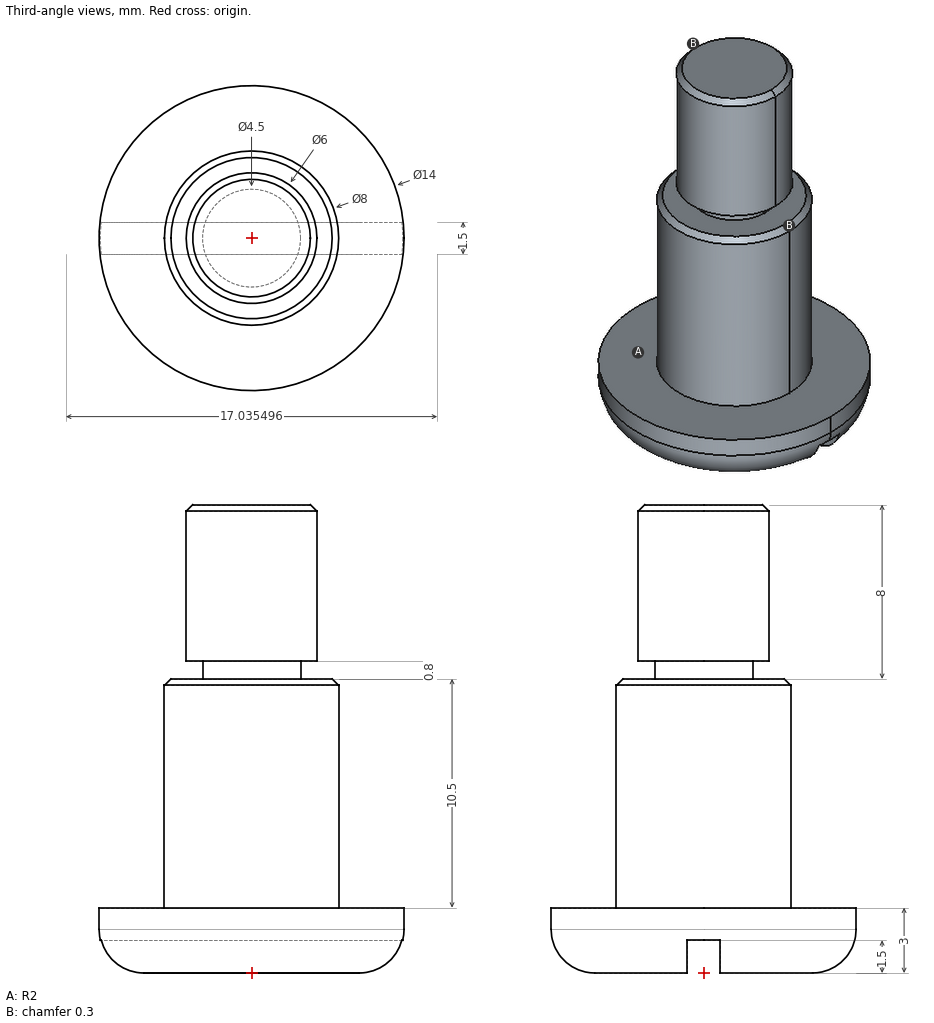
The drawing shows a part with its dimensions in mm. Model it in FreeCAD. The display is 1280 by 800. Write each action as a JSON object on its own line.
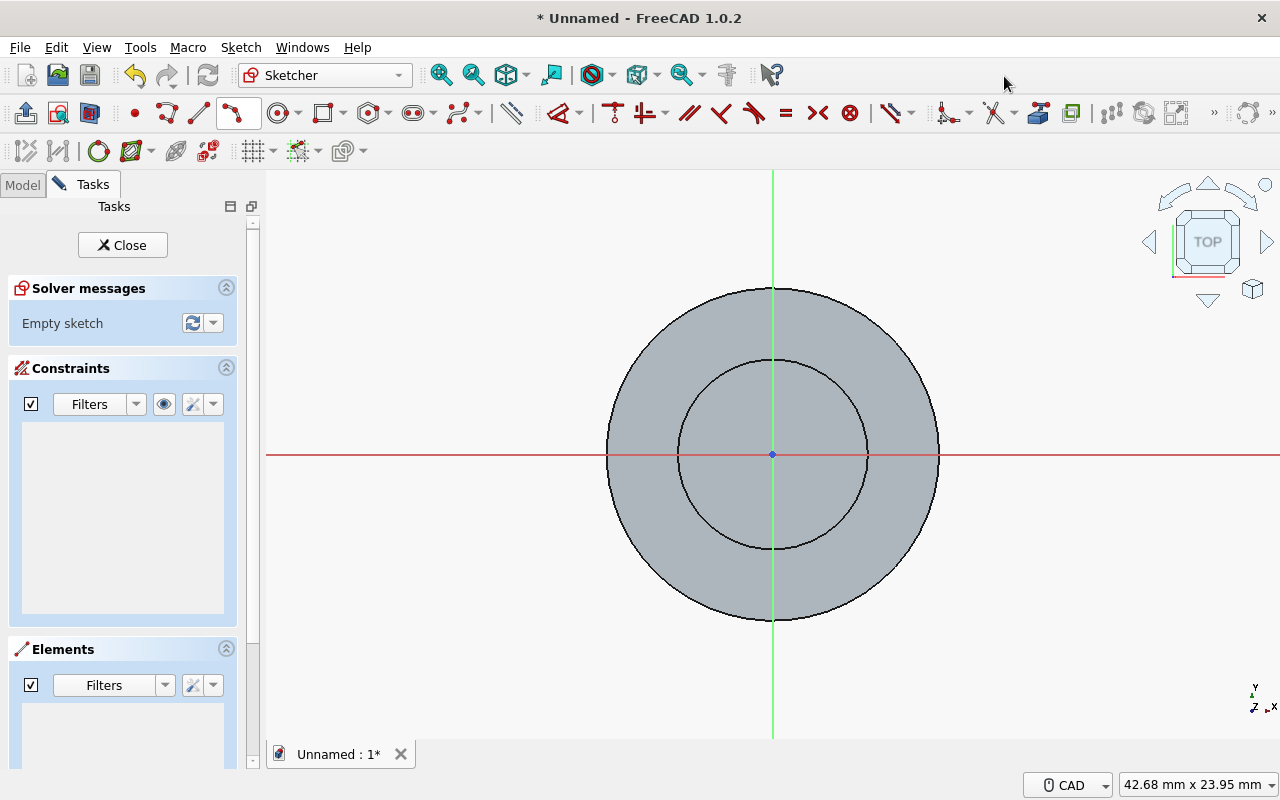
{"action": "scroll", "coordinate": [813, 454], "scroll_direction": "up", "scroll_amount": 5}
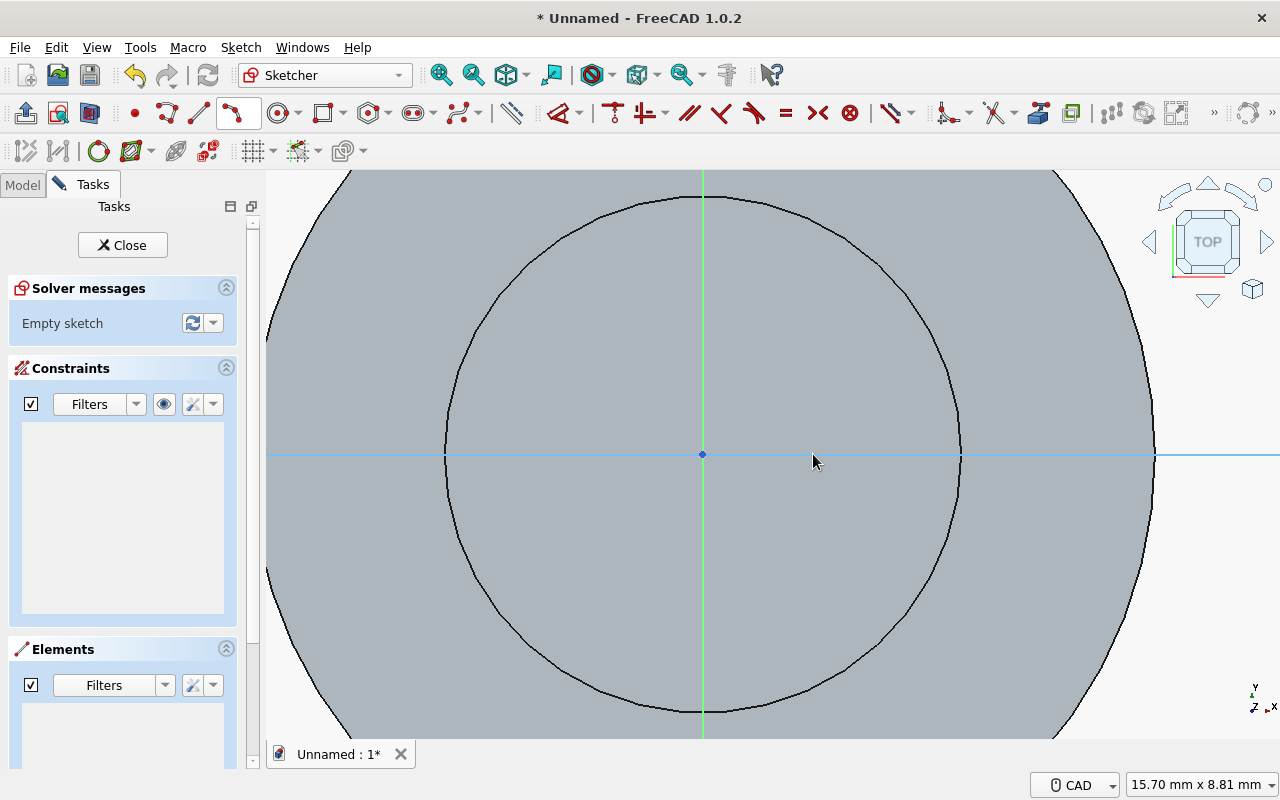
{"action": "left_click", "coordinate": [278, 114]}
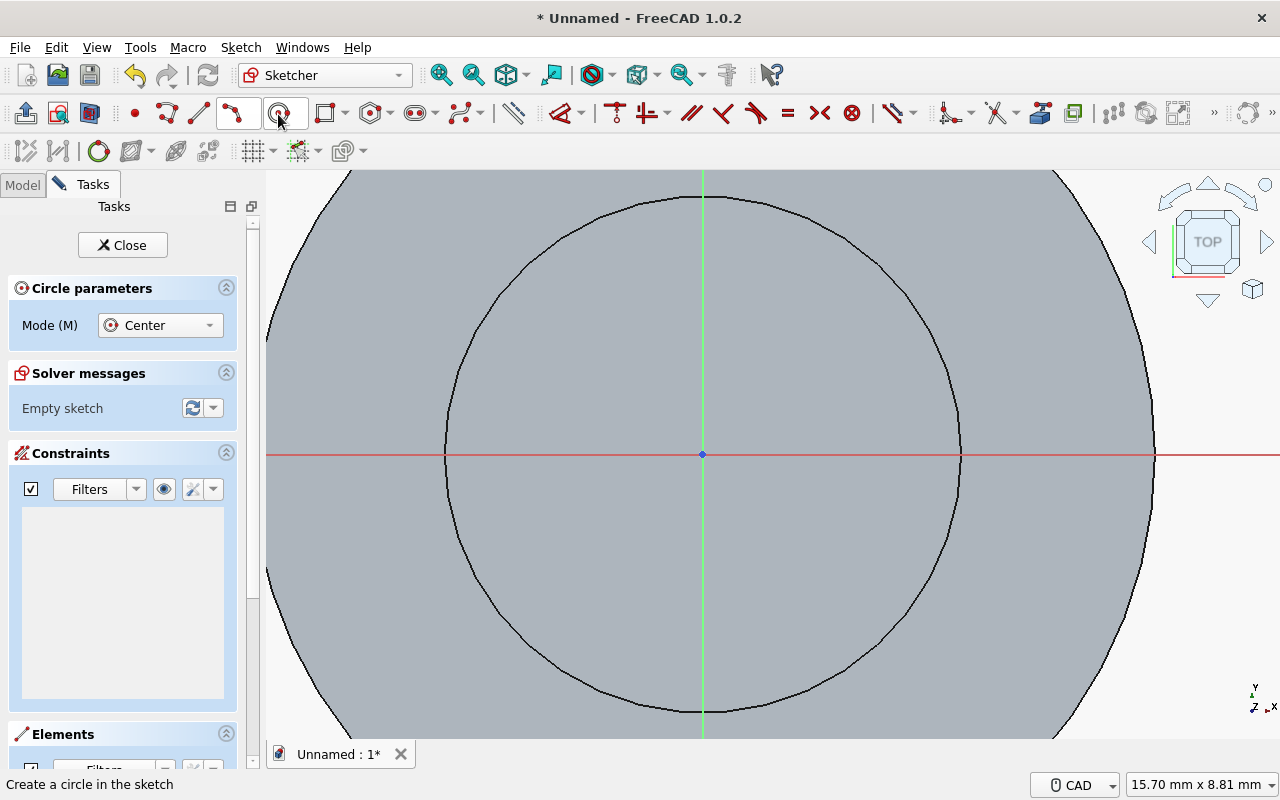
{"action": "left_click", "coordinate": [703, 454]}
{"action": "left_click", "coordinate": [840, 318]}
{"action": "key", "text": "Escape"}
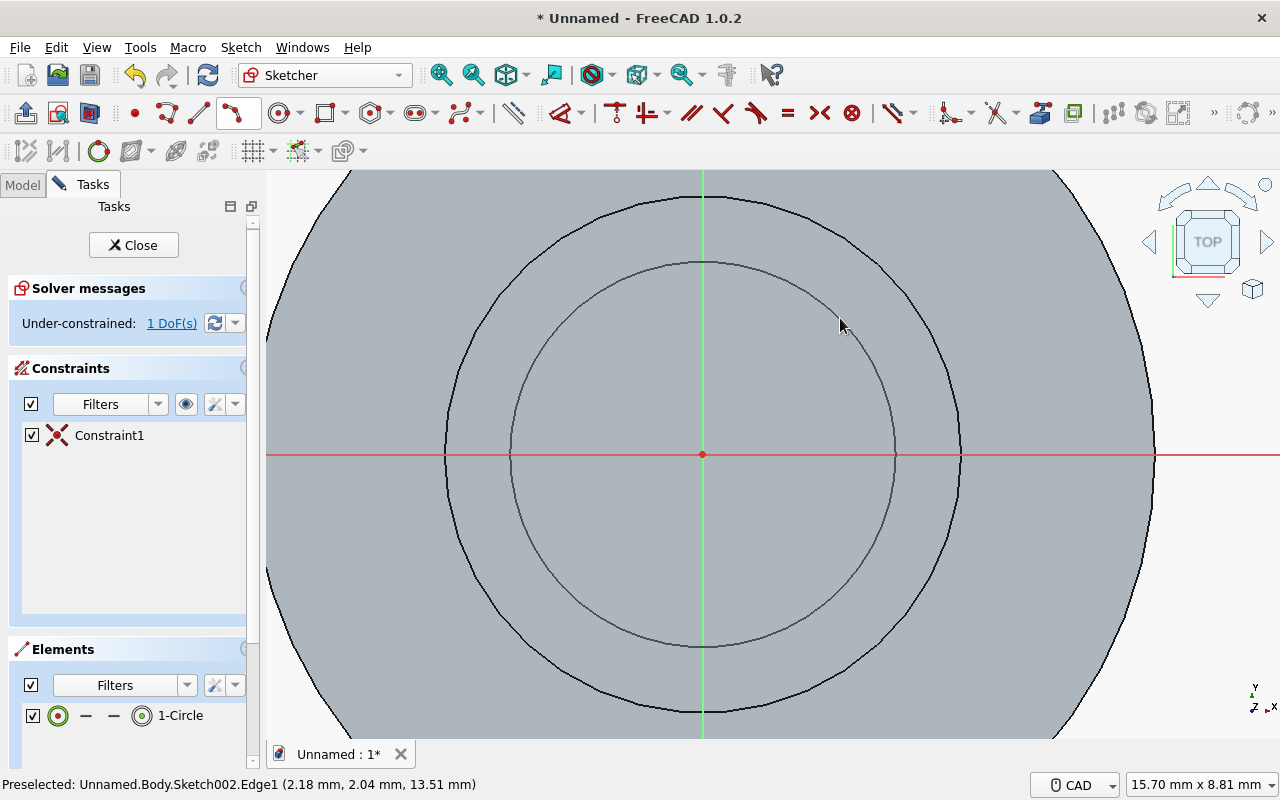
{"action": "key", "text": "d"}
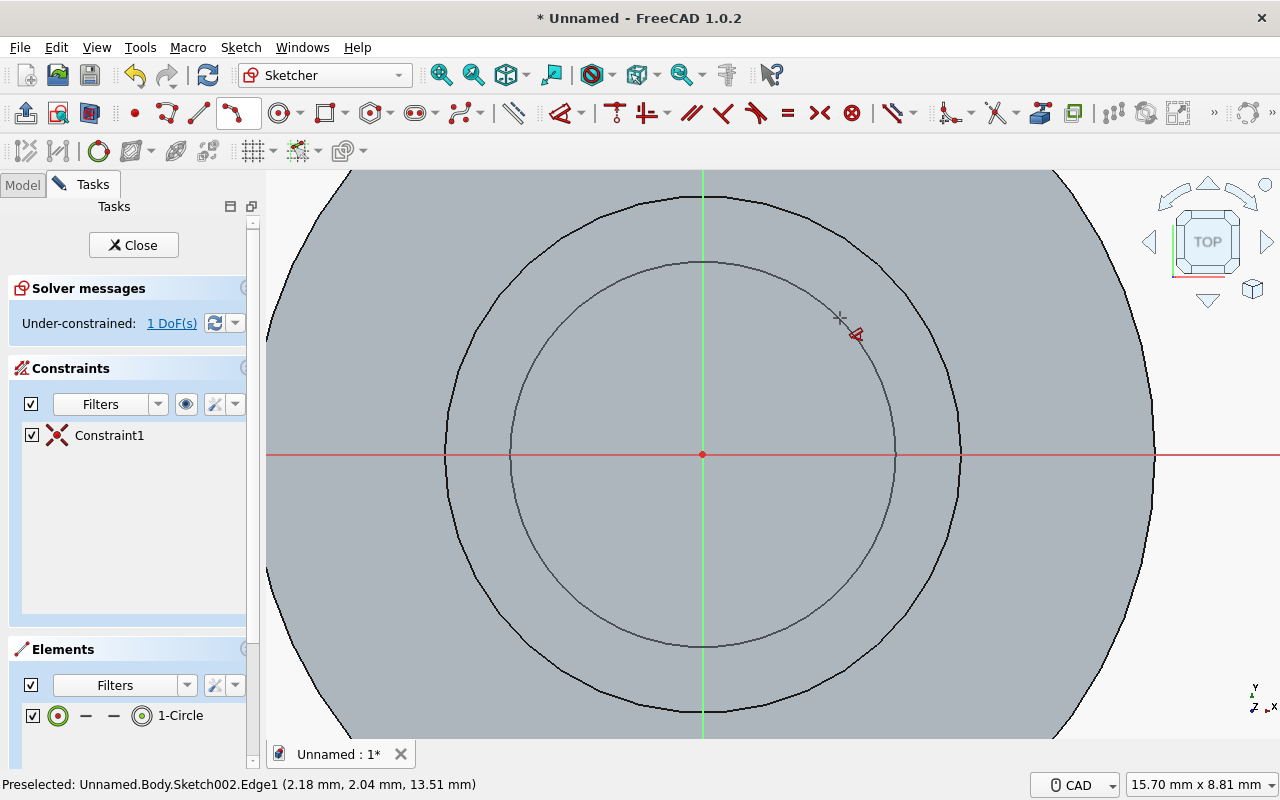
{"action": "left_click", "coordinate": [839, 318]}
{"action": "left_click", "coordinate": [862, 295]}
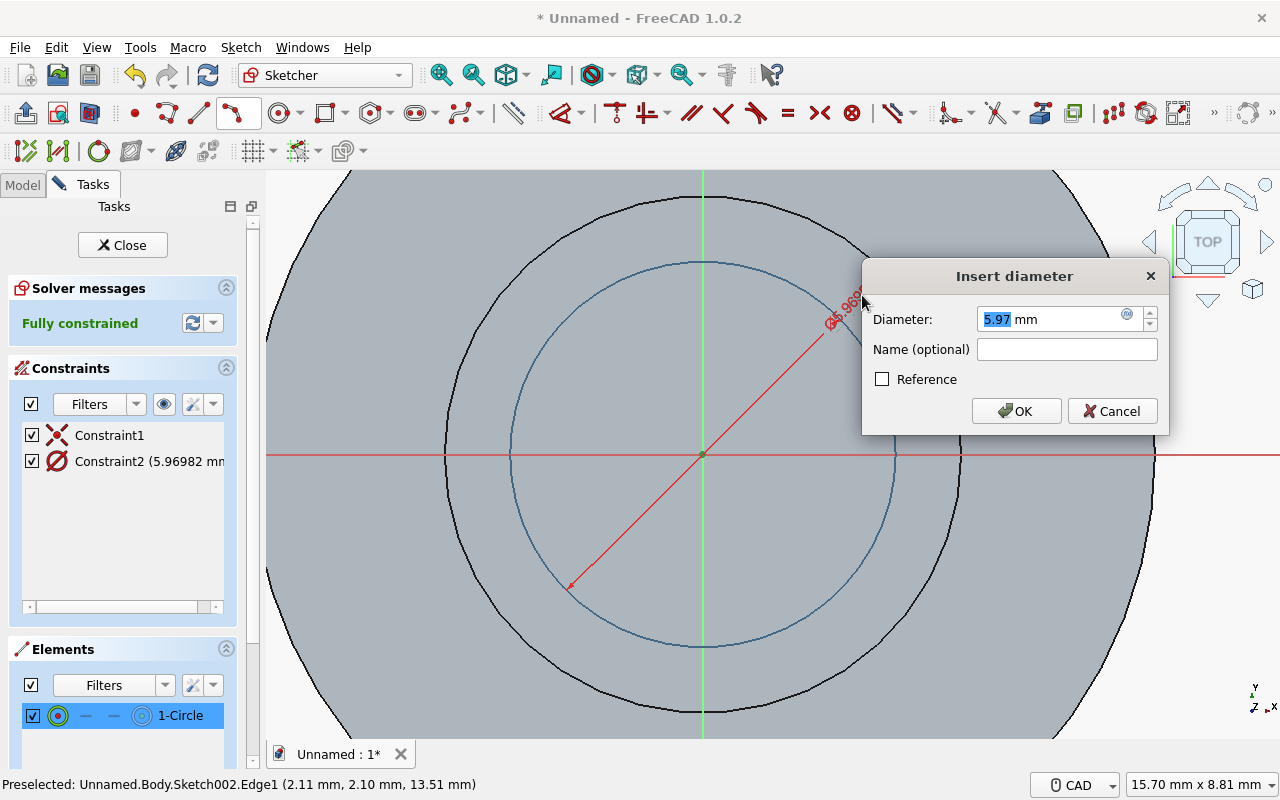
{"action": "type", "text": "6"}
{"action": "key", "text": "Return"}
{"action": "key", "text": "Escape"}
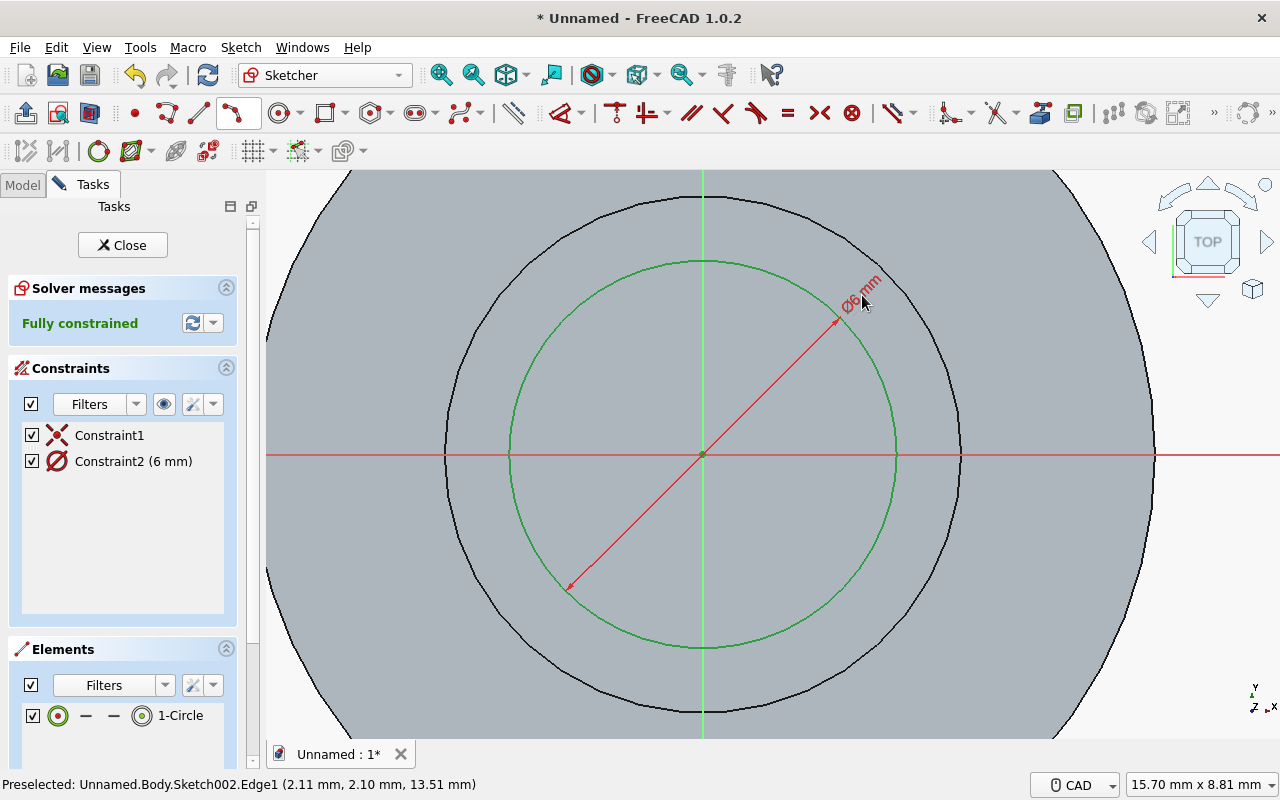
{"action": "left_click", "coordinate": [123, 245]}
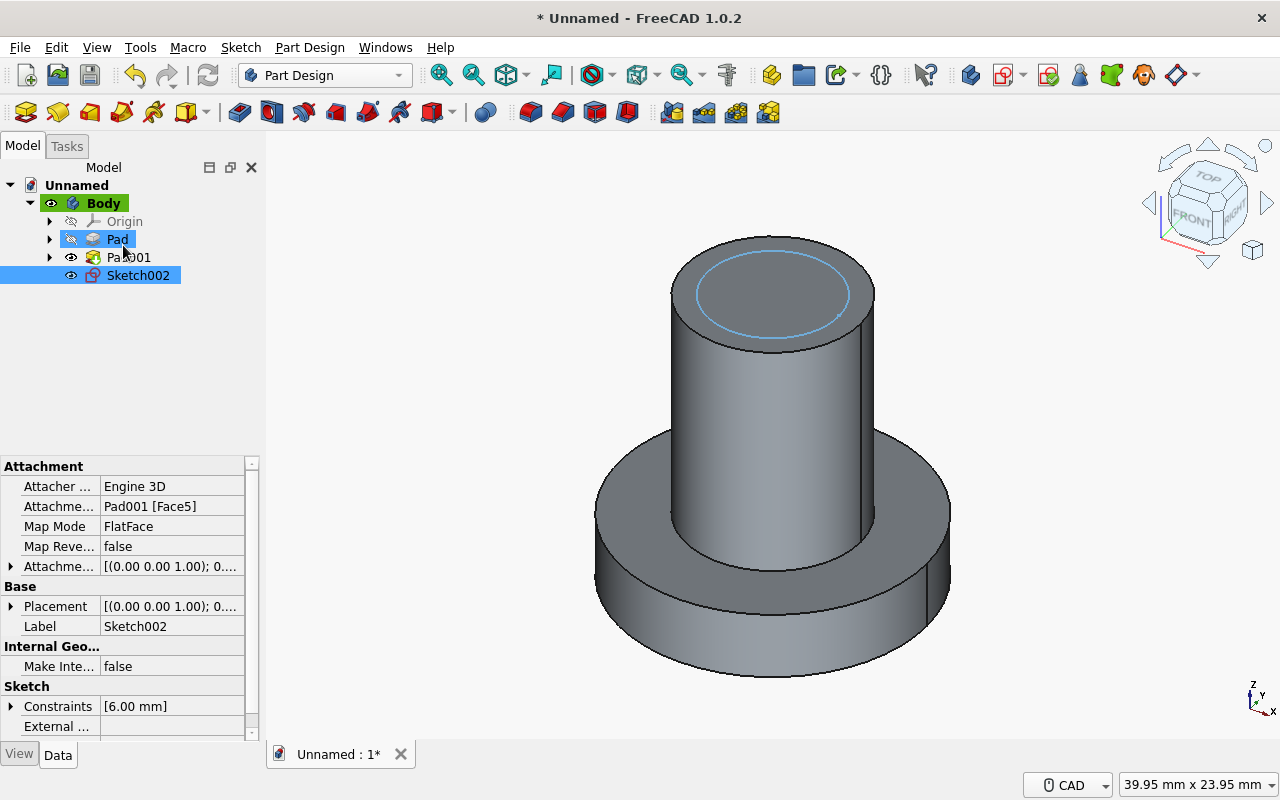
{"action": "left_click", "coordinate": [26, 112]}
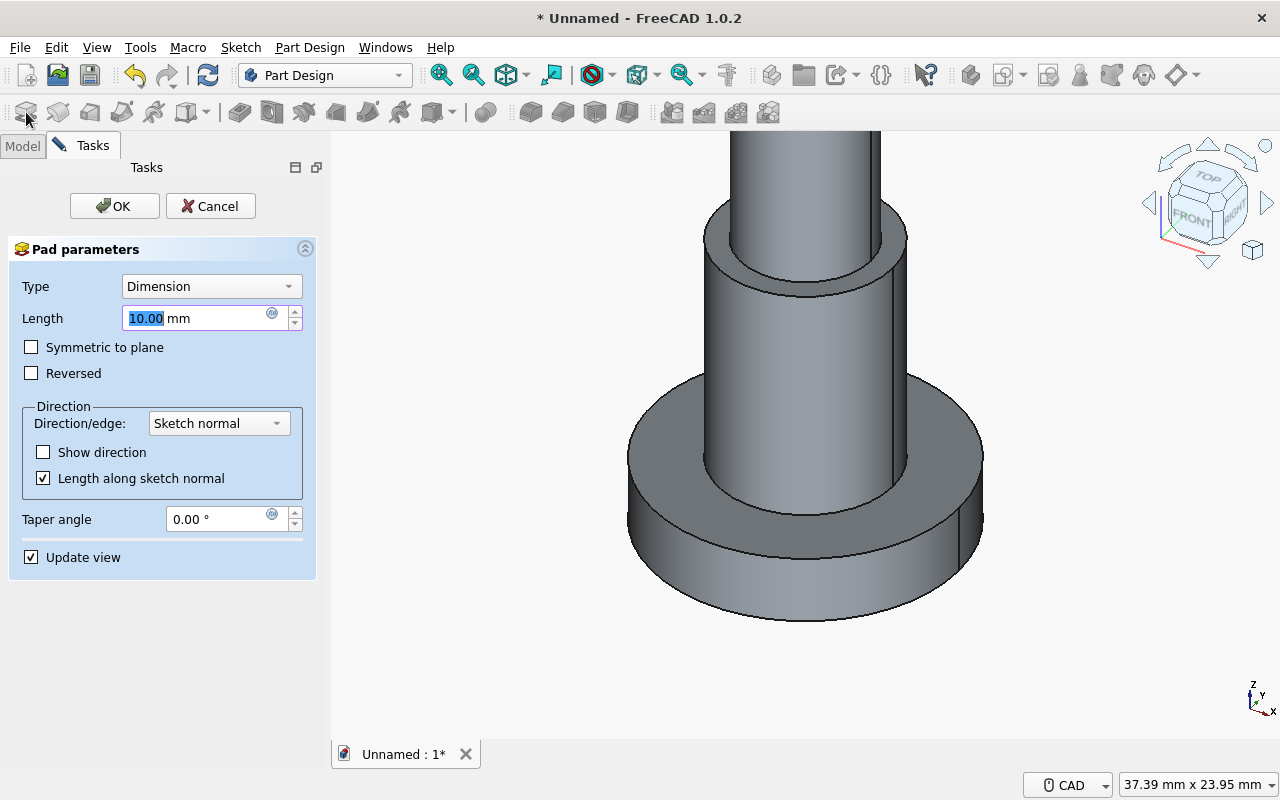
{"action": "type", "text": "8"}
{"action": "key", "text": "Tab"}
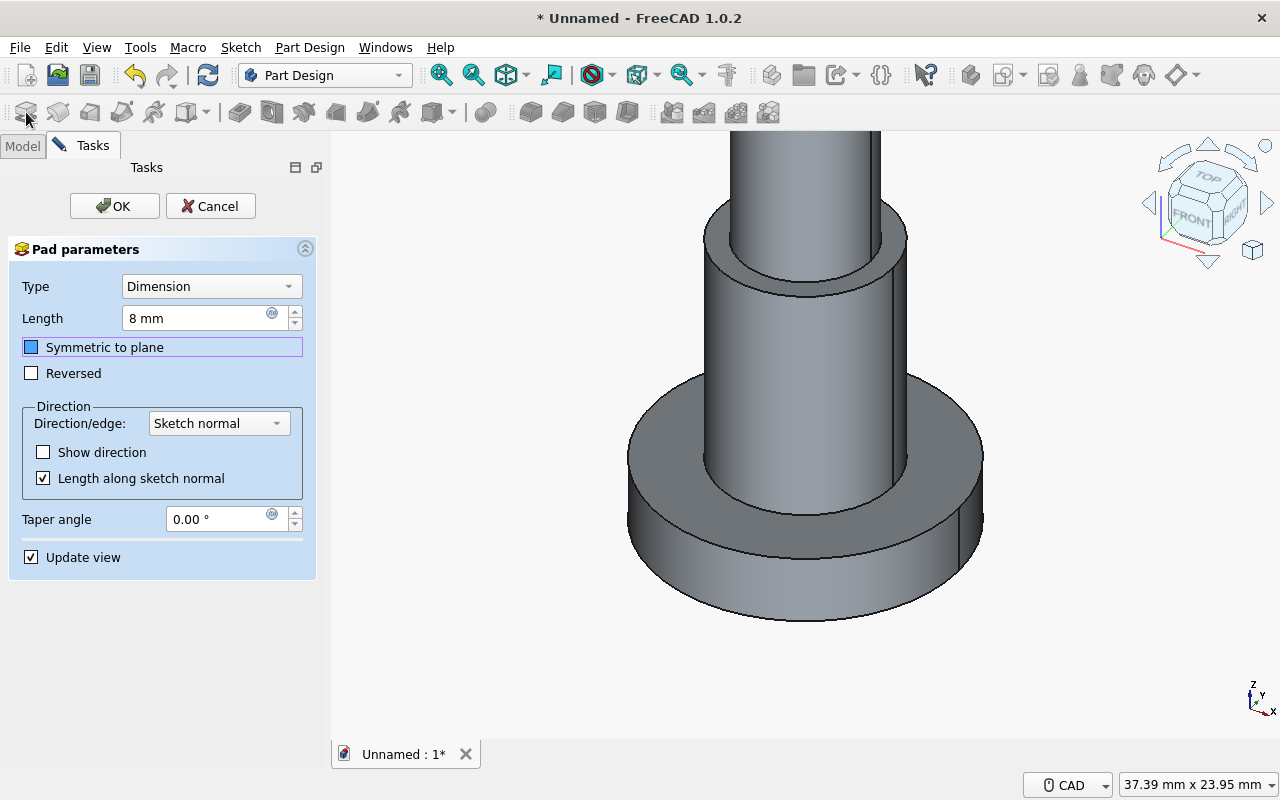
{"action": "left_click", "coordinate": [115, 206]}